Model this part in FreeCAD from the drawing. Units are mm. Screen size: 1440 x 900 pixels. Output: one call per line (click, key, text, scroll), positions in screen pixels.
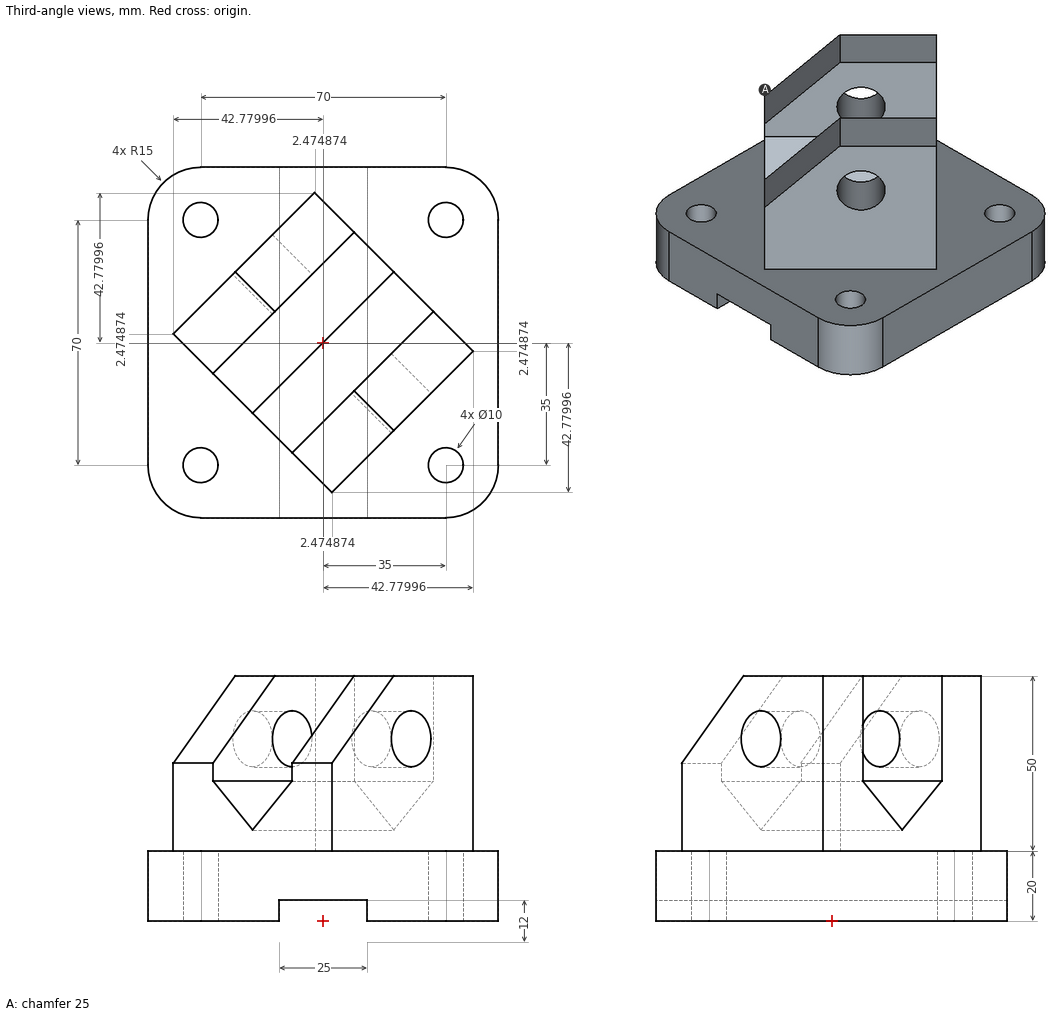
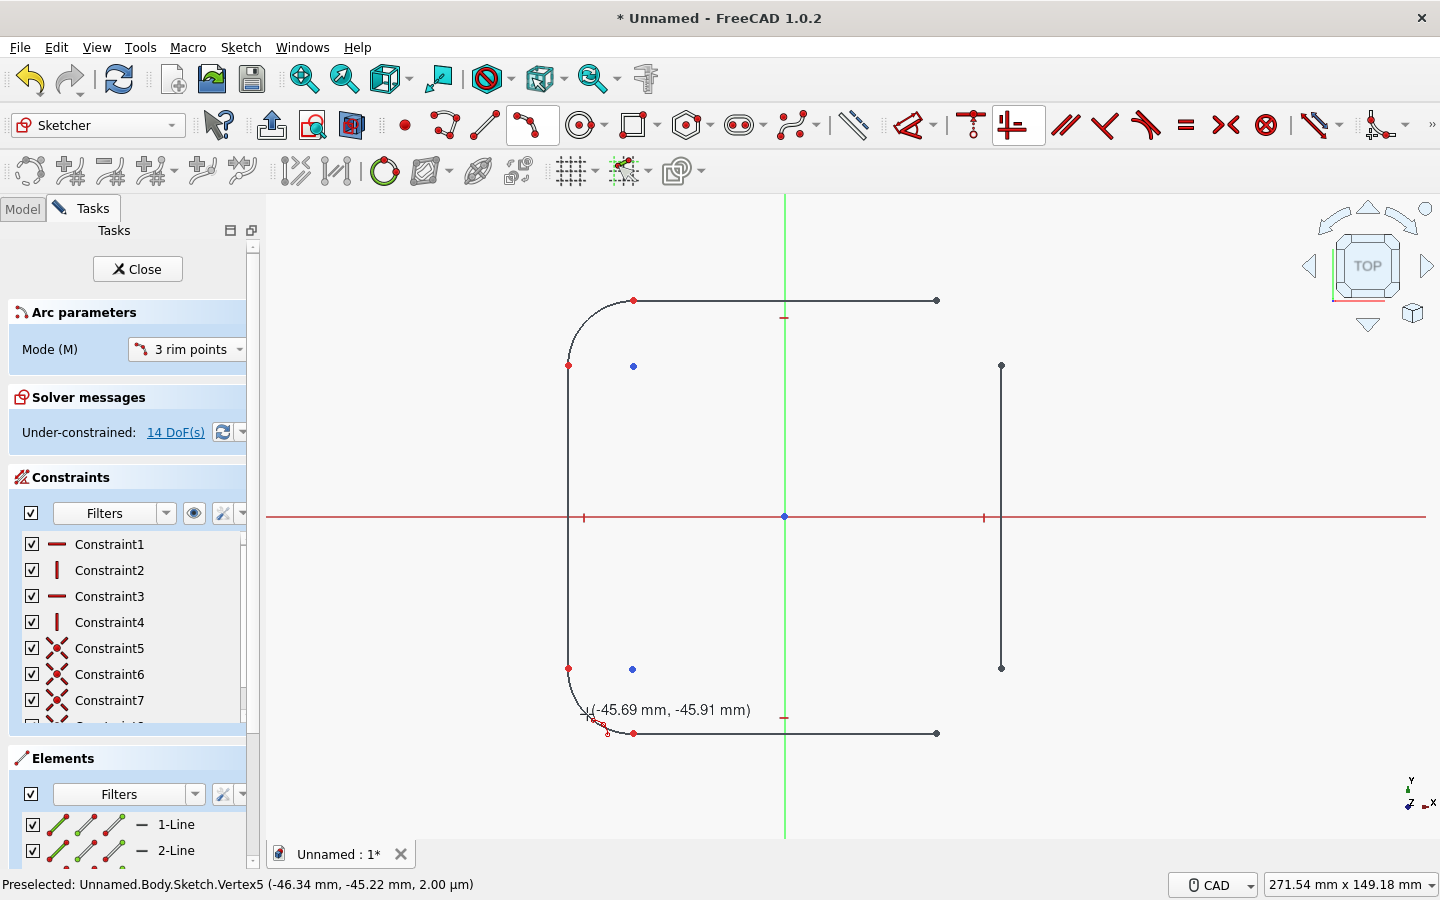
click(936, 734)
click(1001, 669)
click(982, 714)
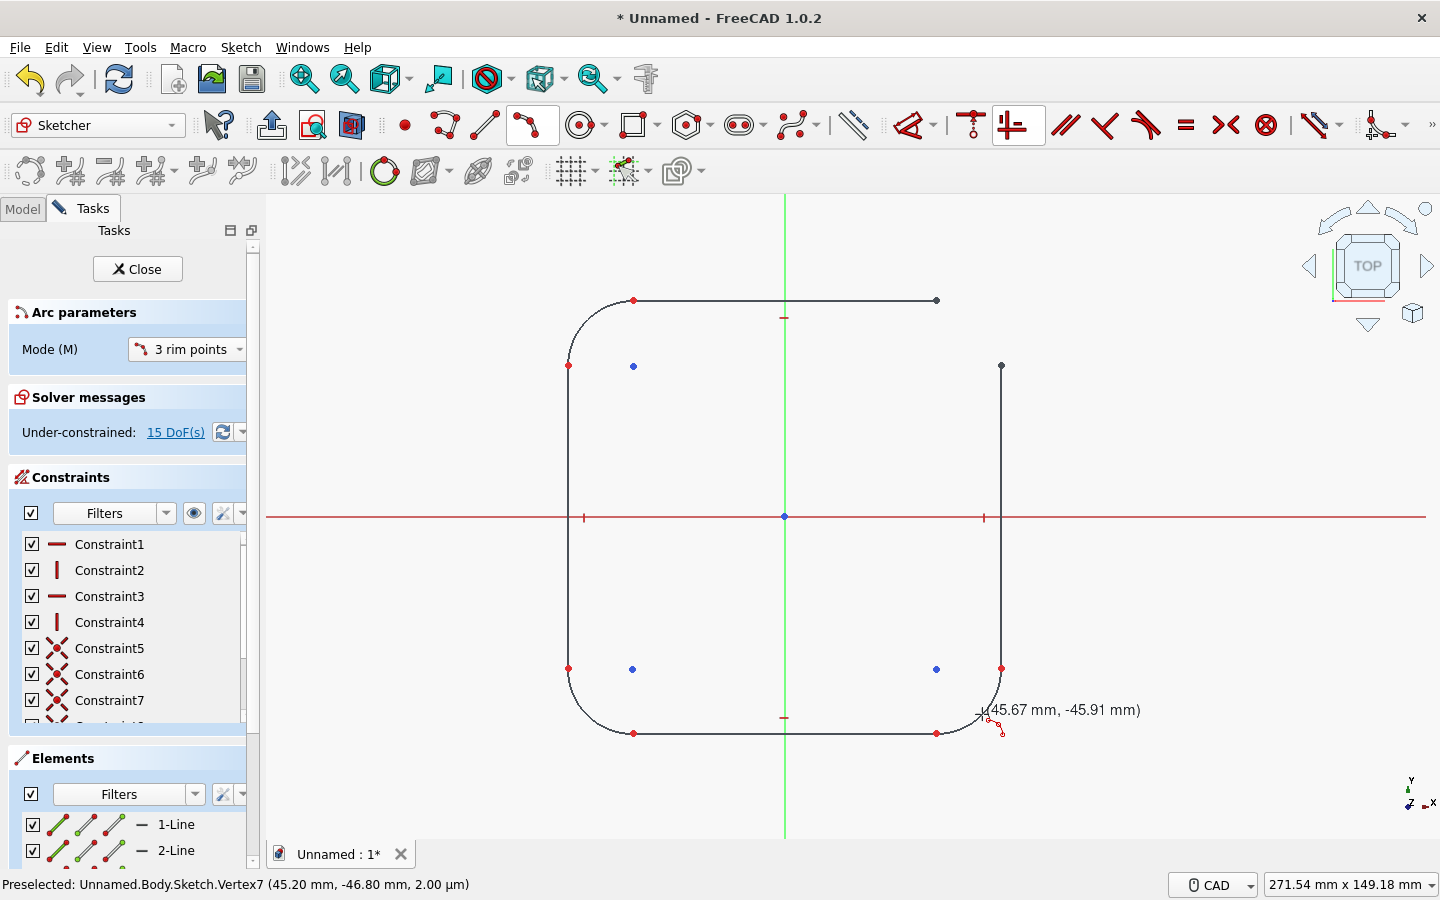
click(1001, 366)
click(936, 301)
click(982, 319)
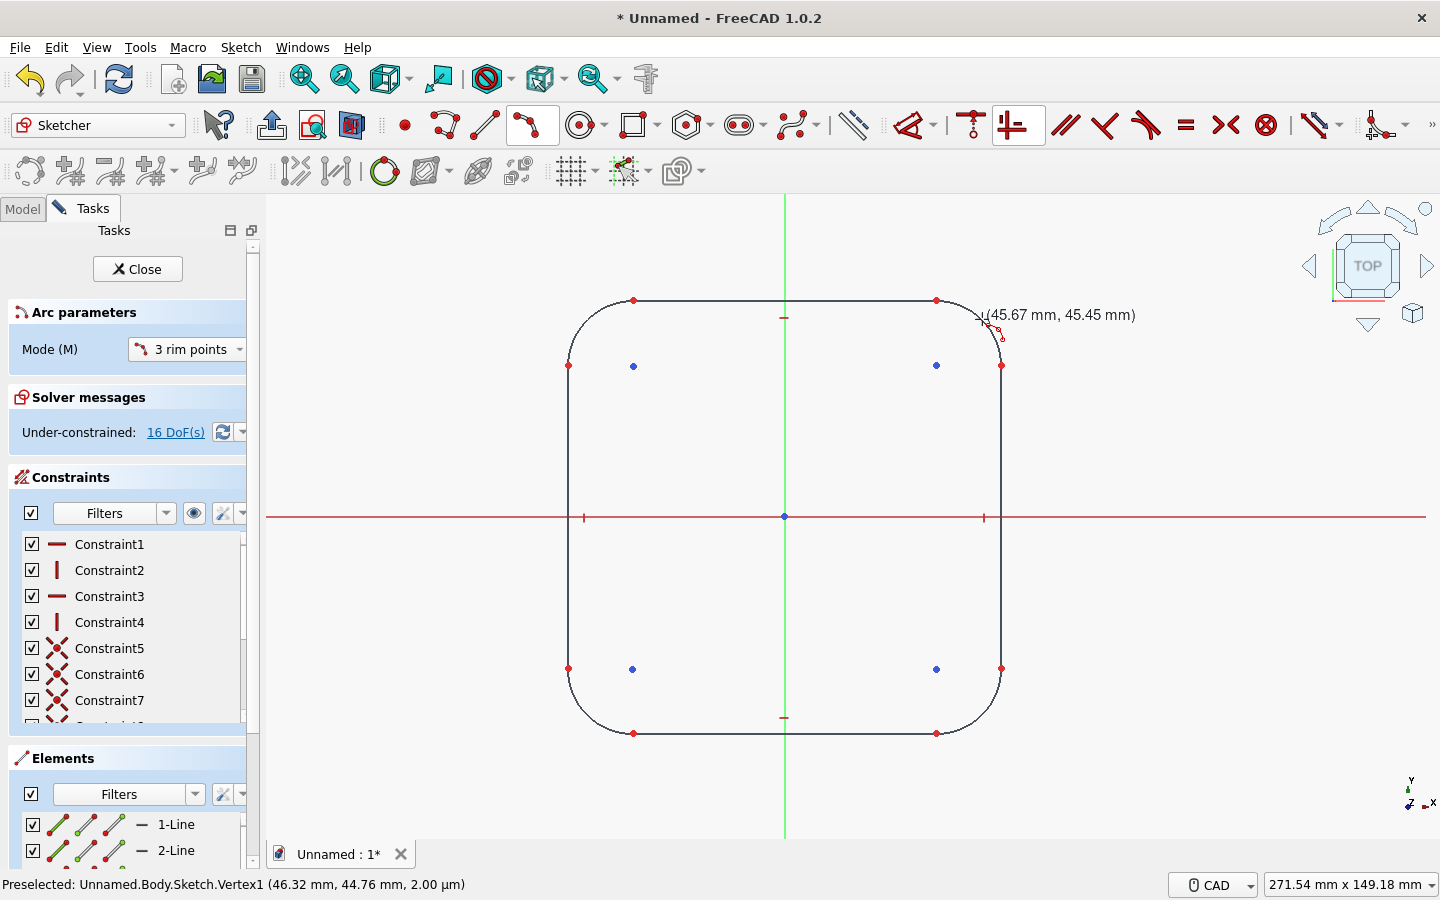
click(580, 126)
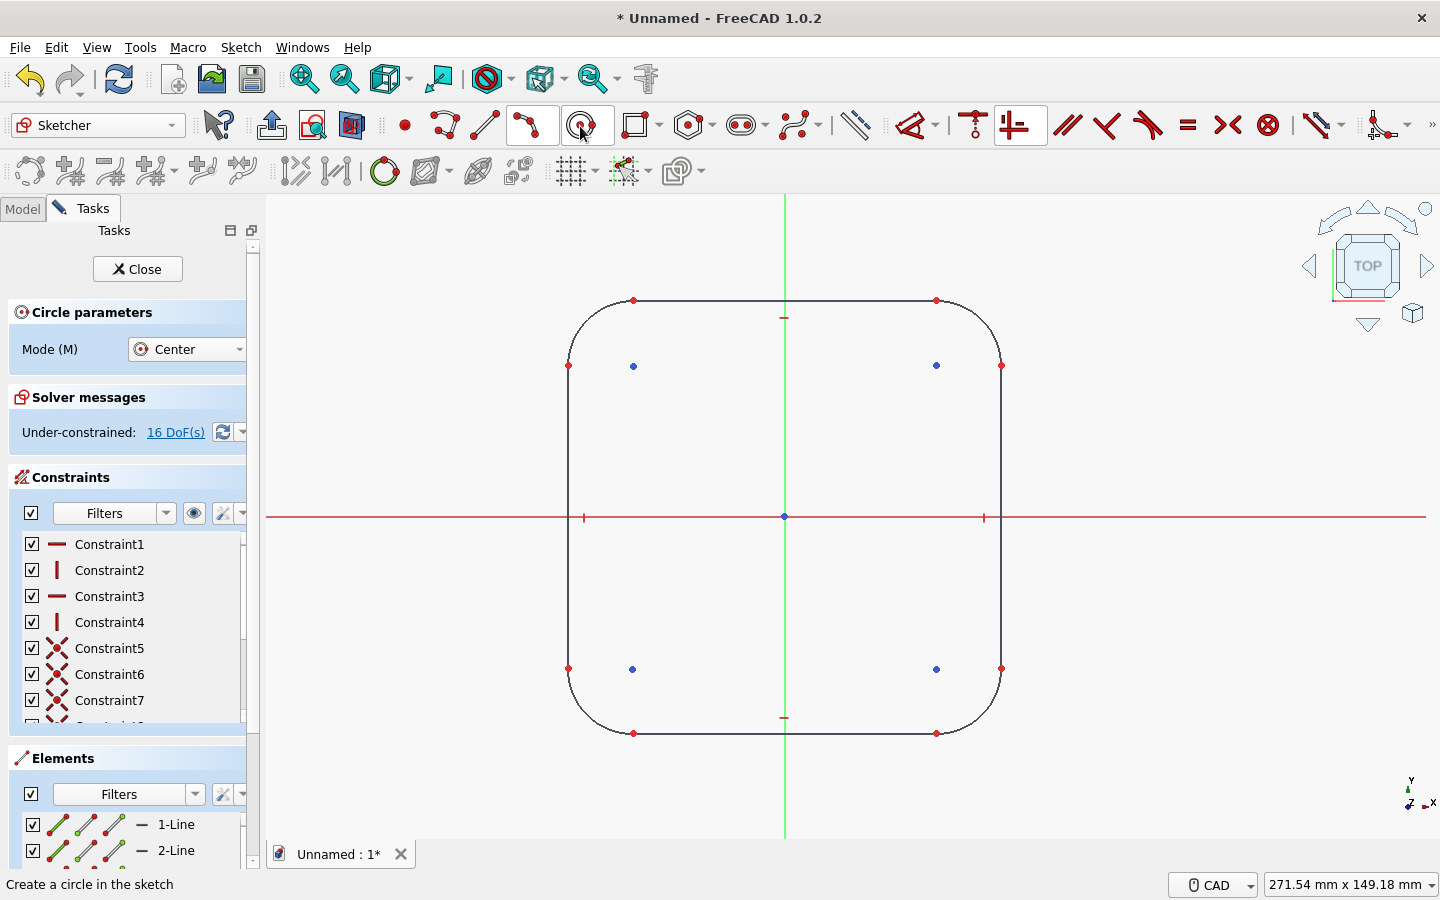
click(936, 668)
move(951, 653)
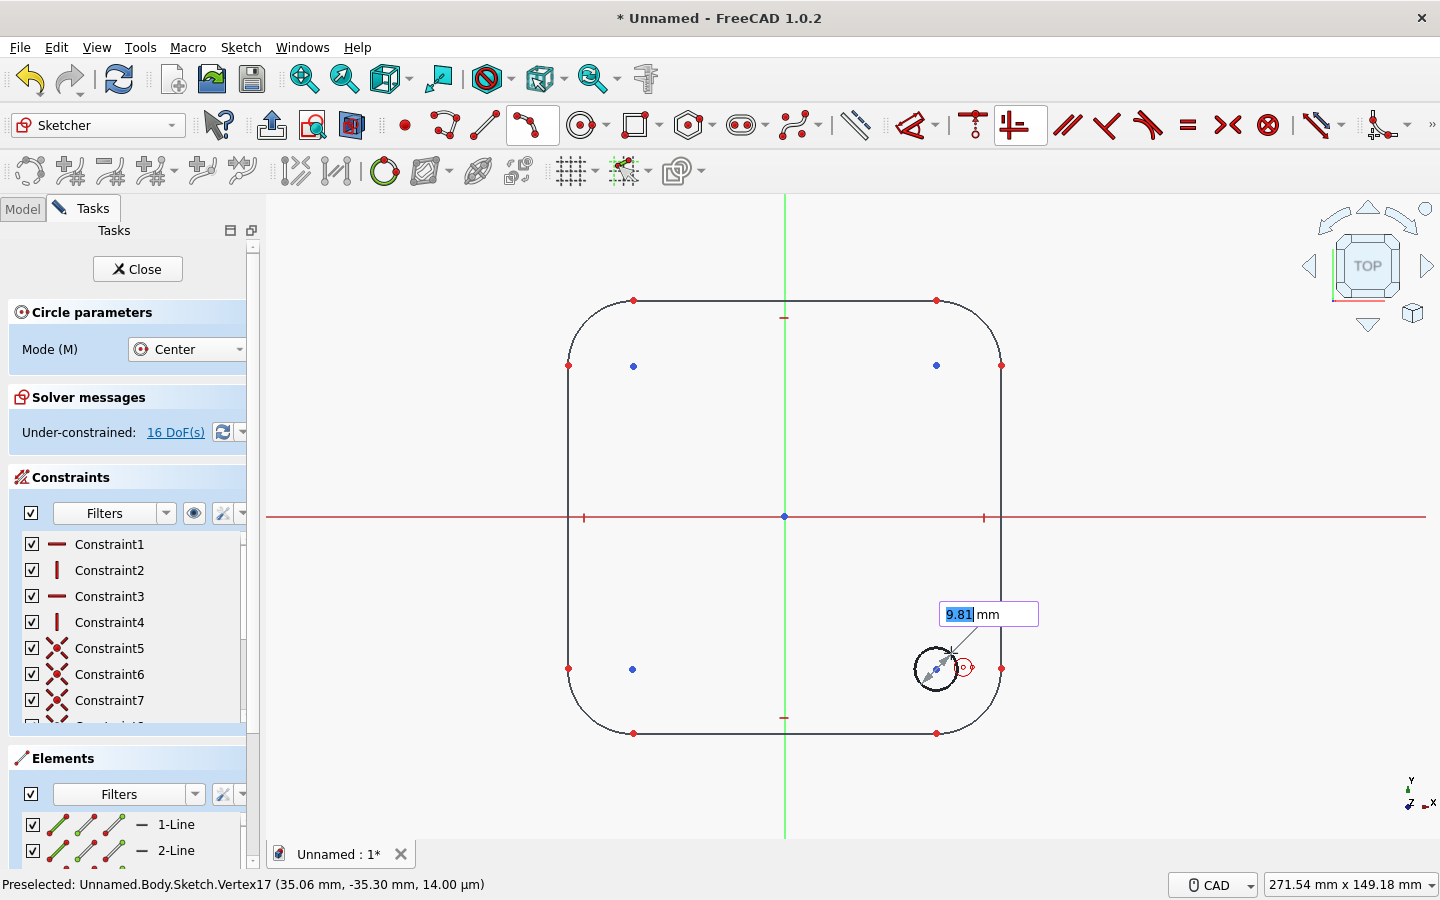
text(10)
key(Return)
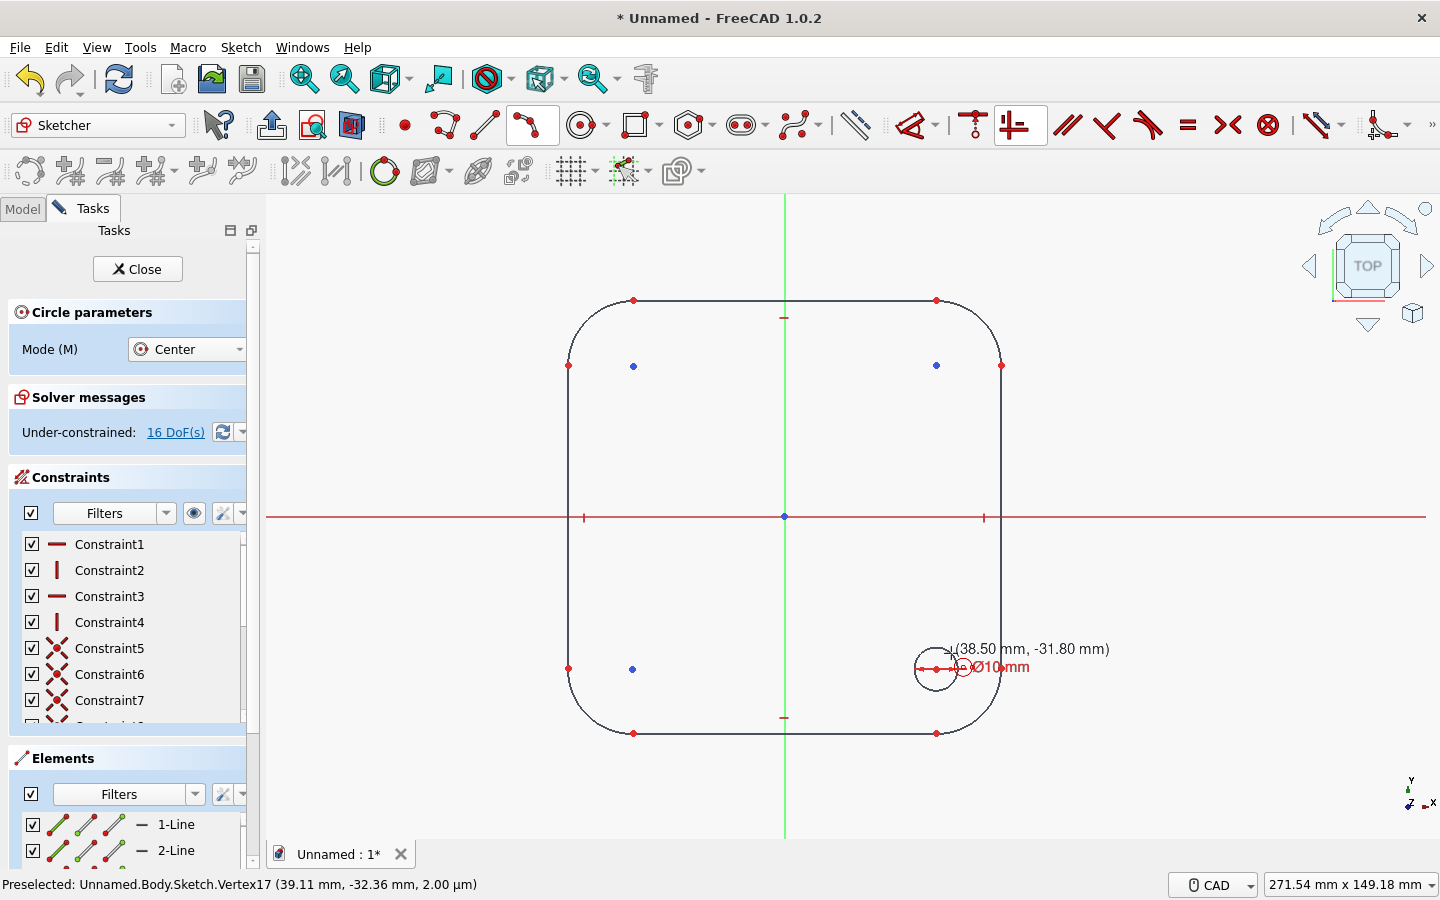
click(633, 668)
move(648, 653)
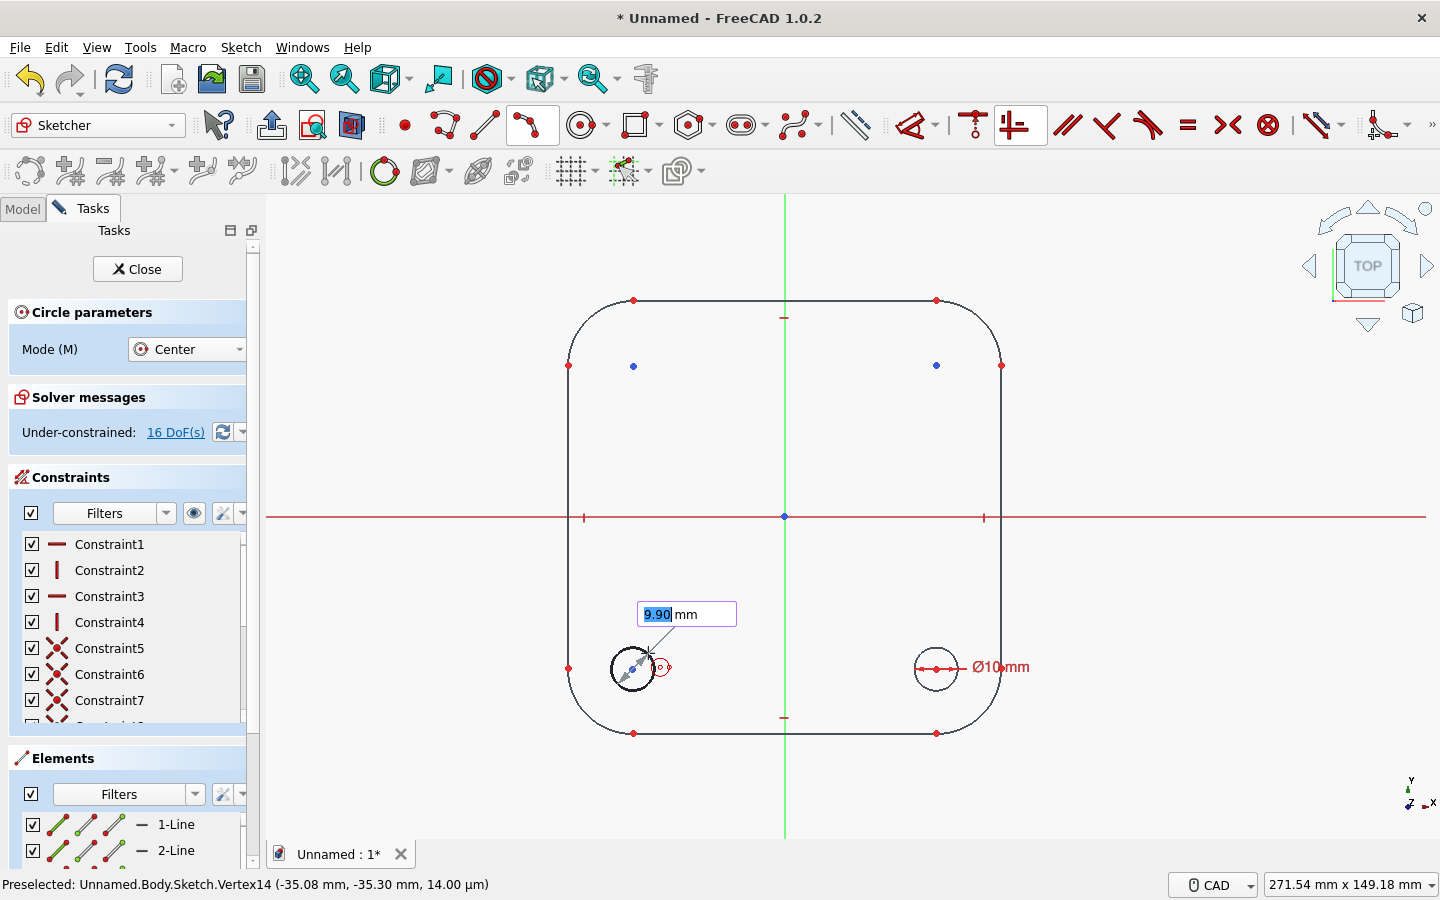
text(10)
key(Return)